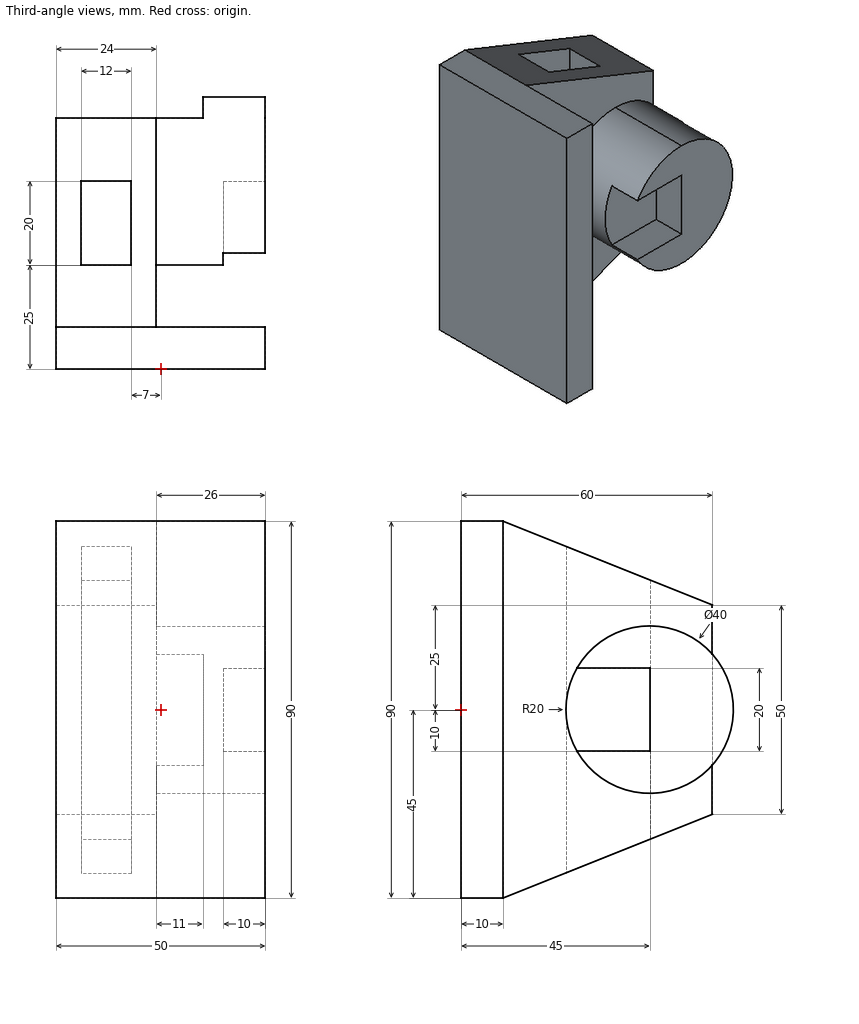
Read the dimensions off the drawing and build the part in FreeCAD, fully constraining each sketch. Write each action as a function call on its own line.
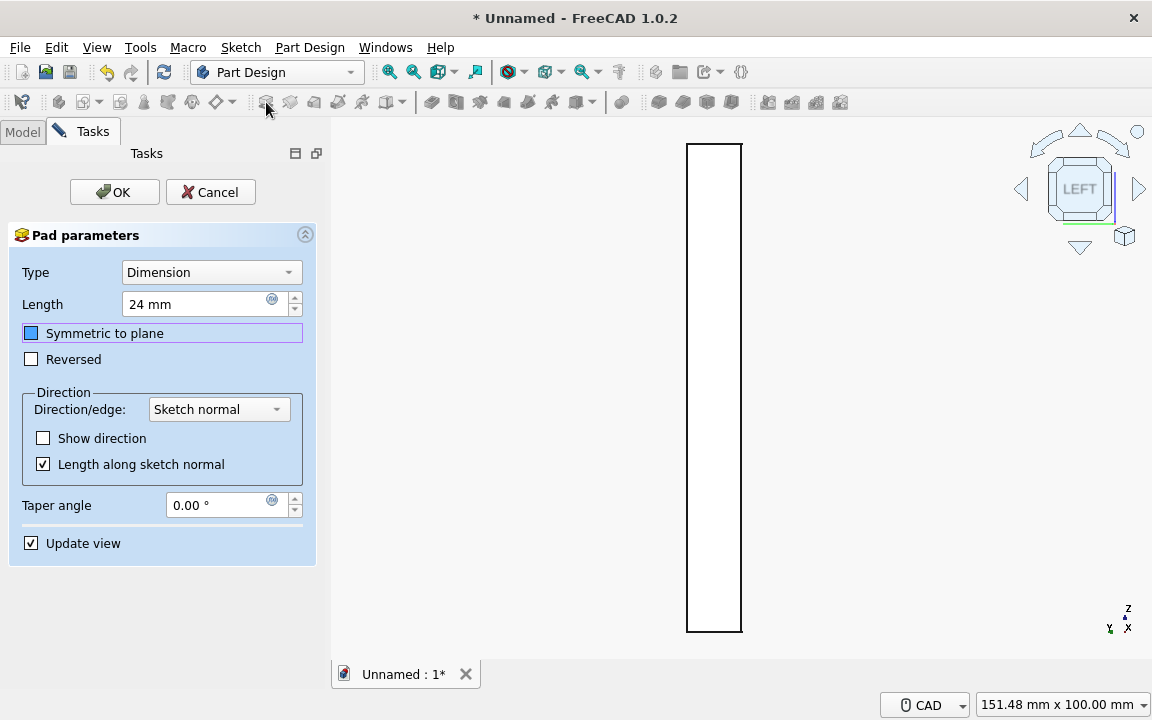
click(30, 359)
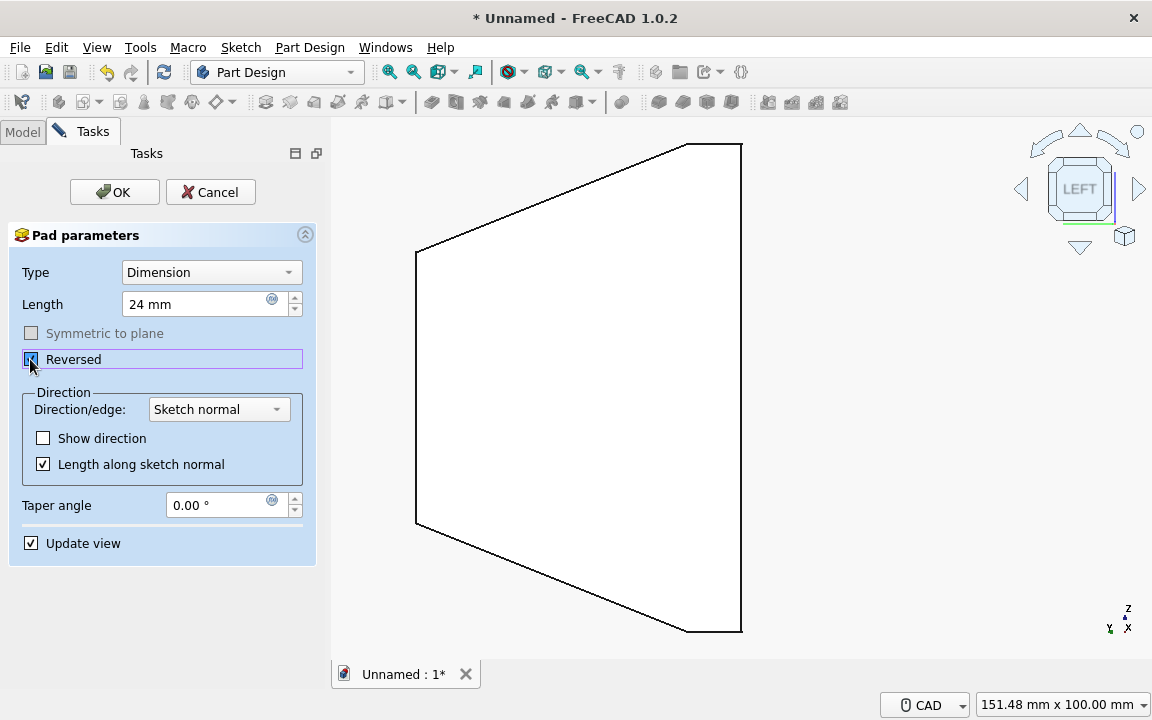
click(115, 192)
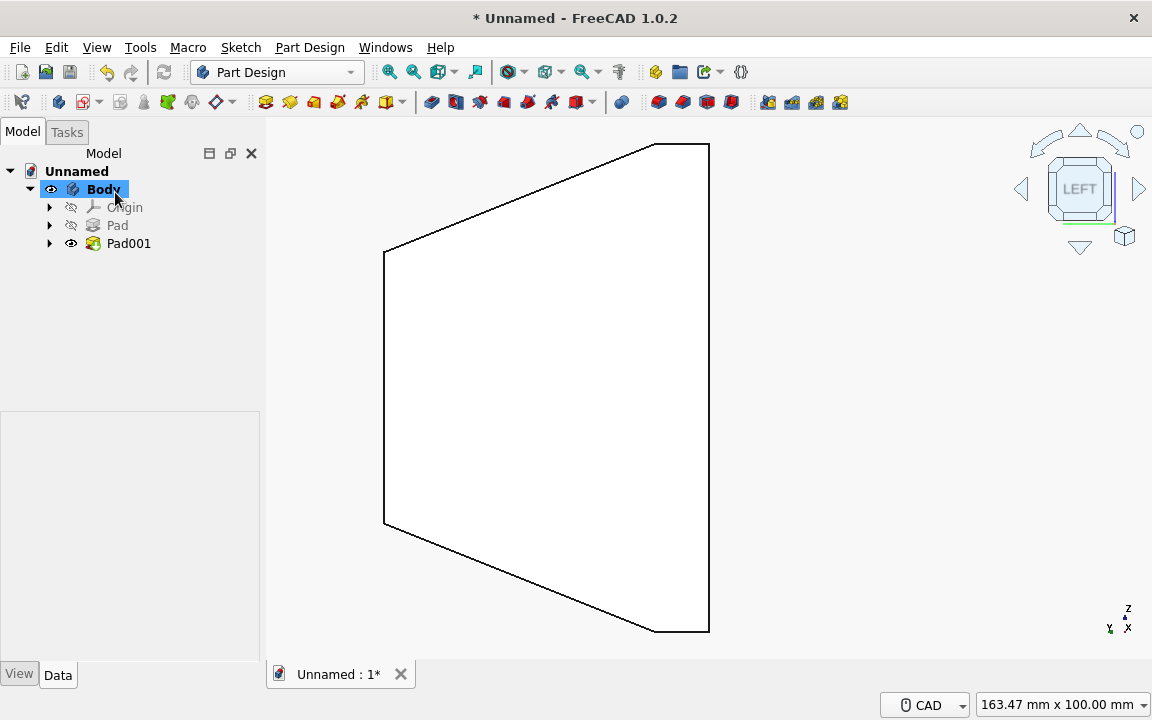
key(5)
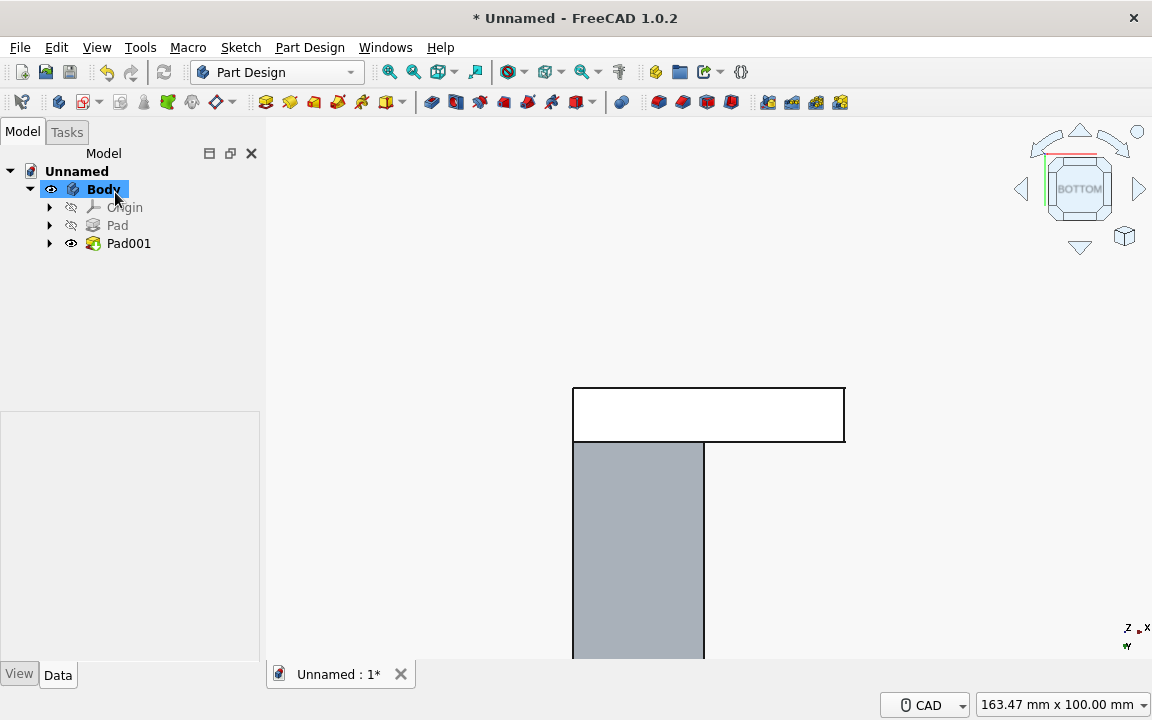
click(390, 72)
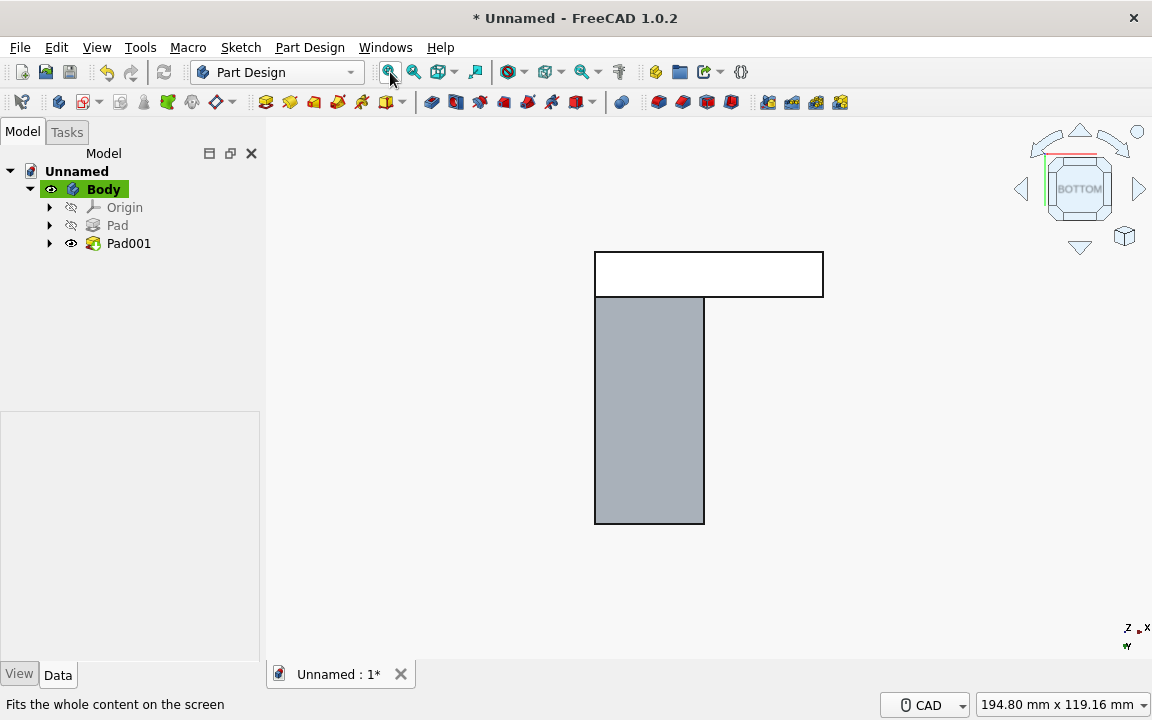
click(774, 273)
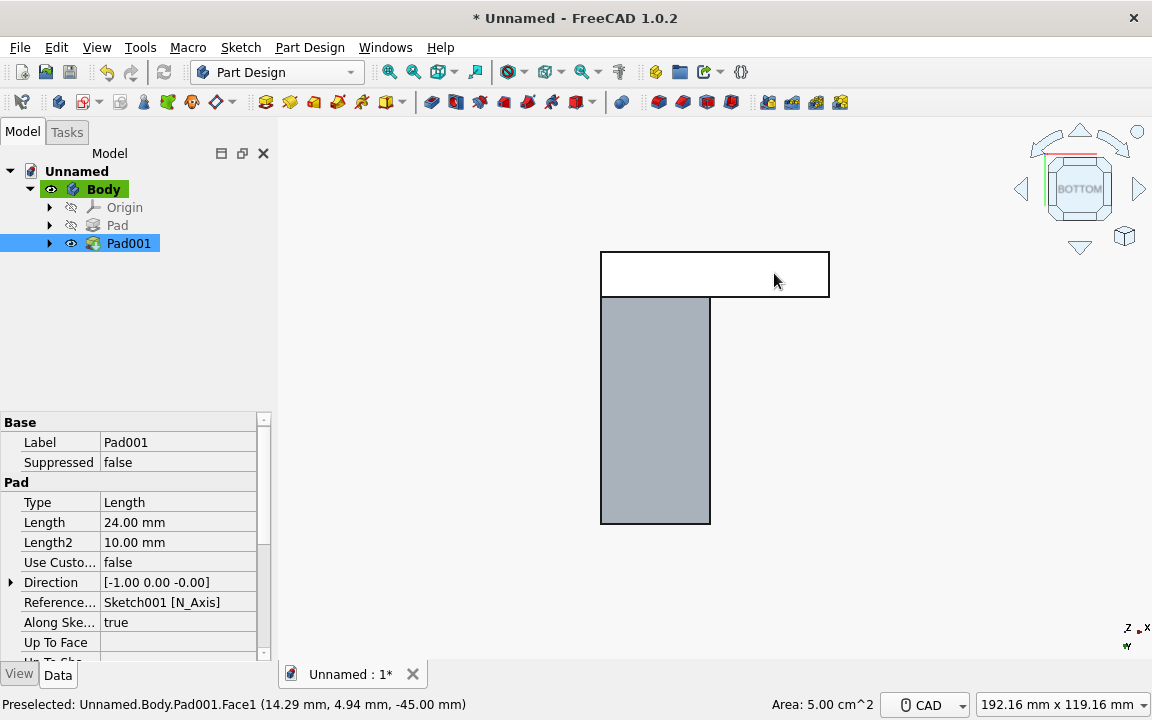
click(84, 102)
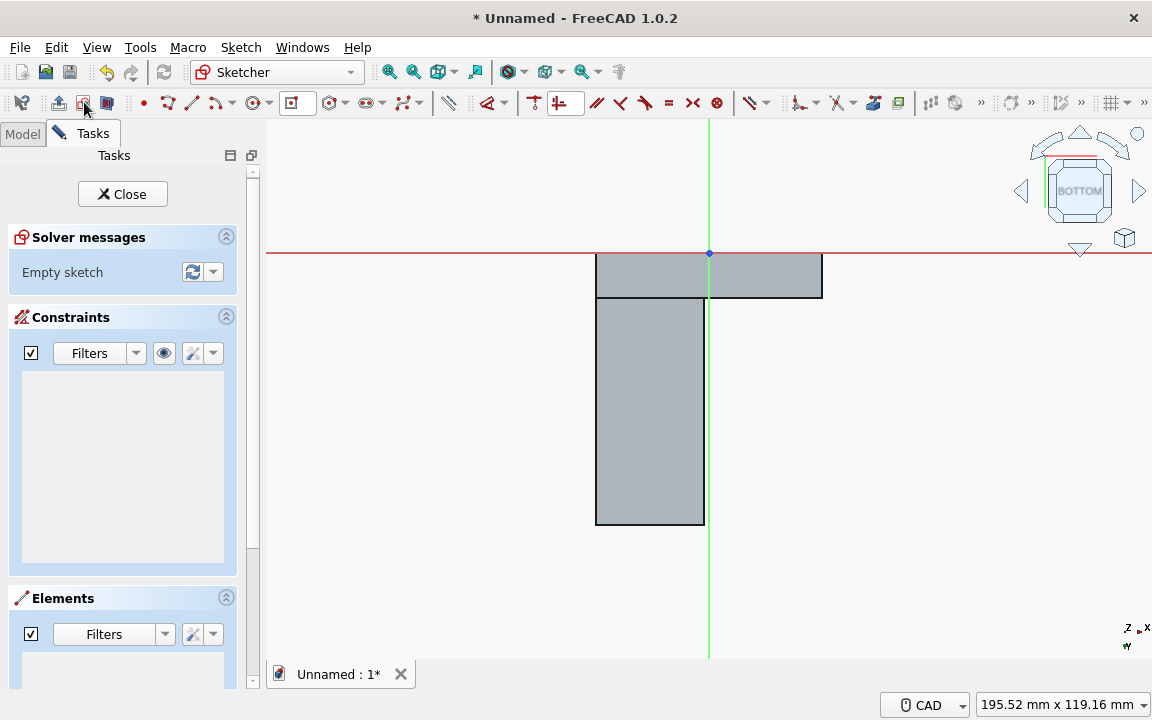
scroll(697, 314, up, 3)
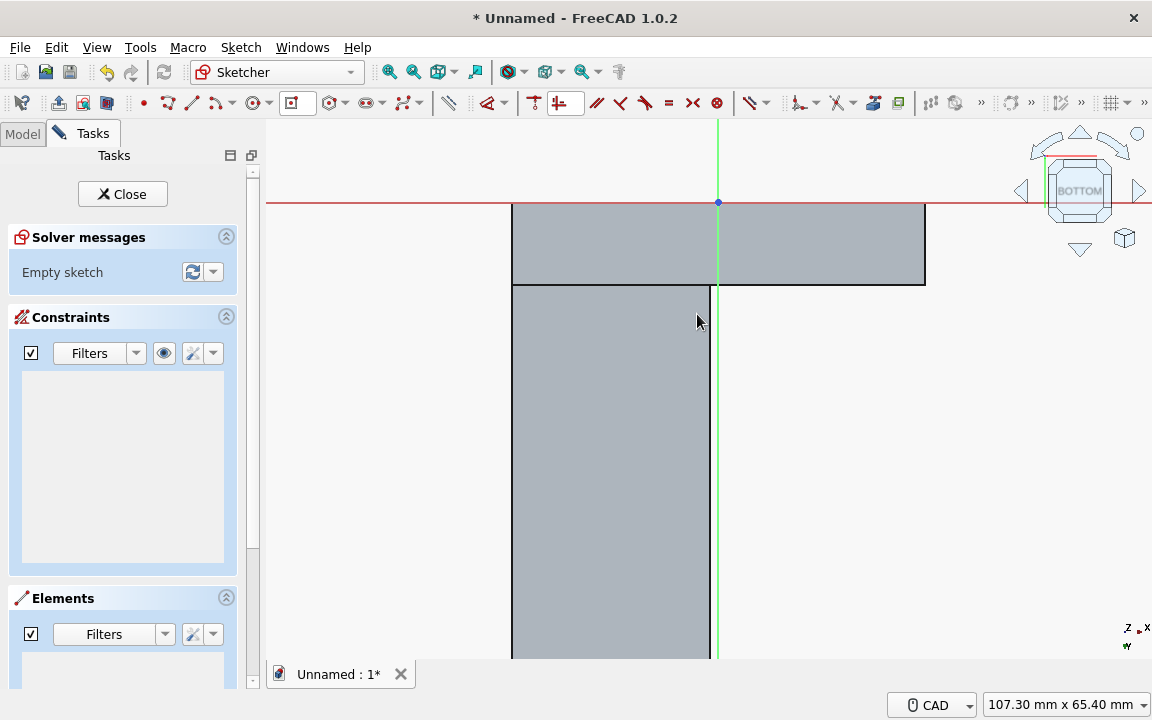
key(g)
key(r)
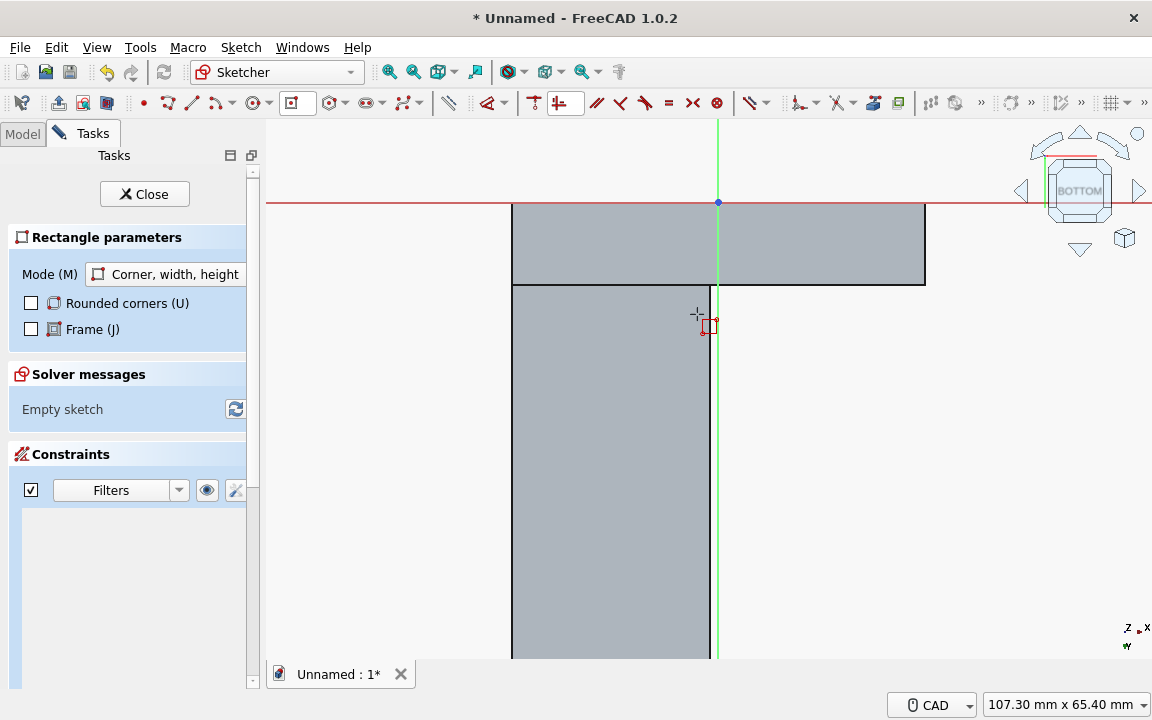
click(562, 409)
move(661, 574)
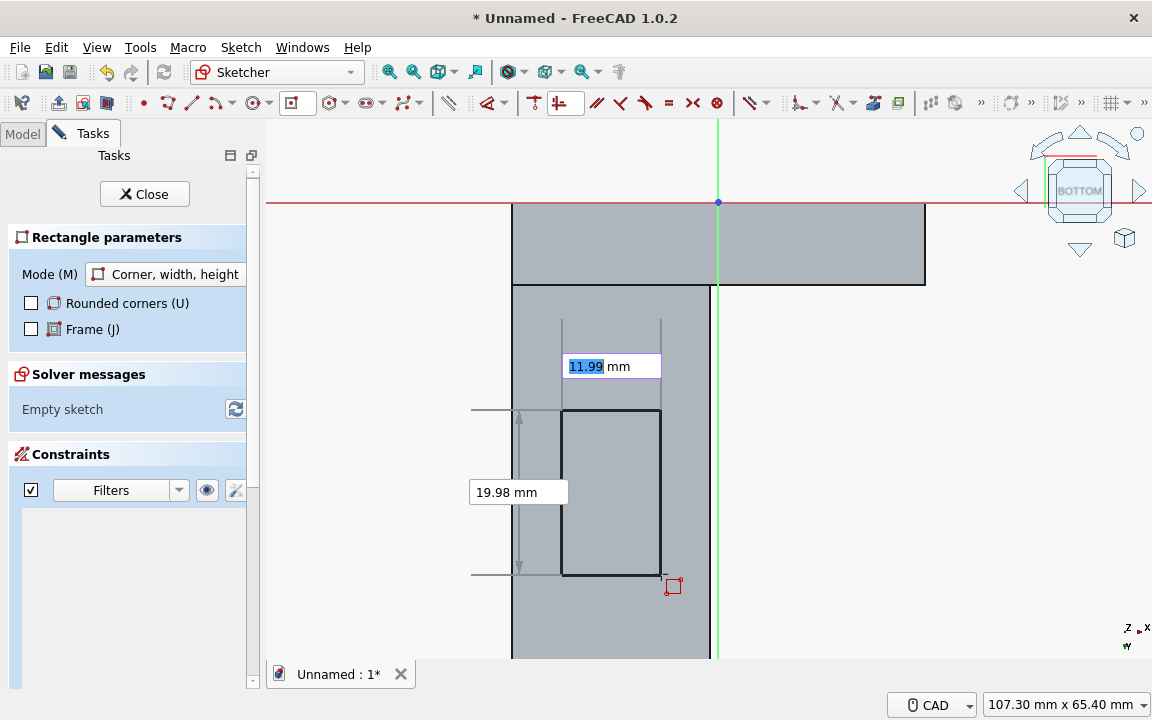
text(12)
key(Tab)
text(20)
key(Return)
key(Escape)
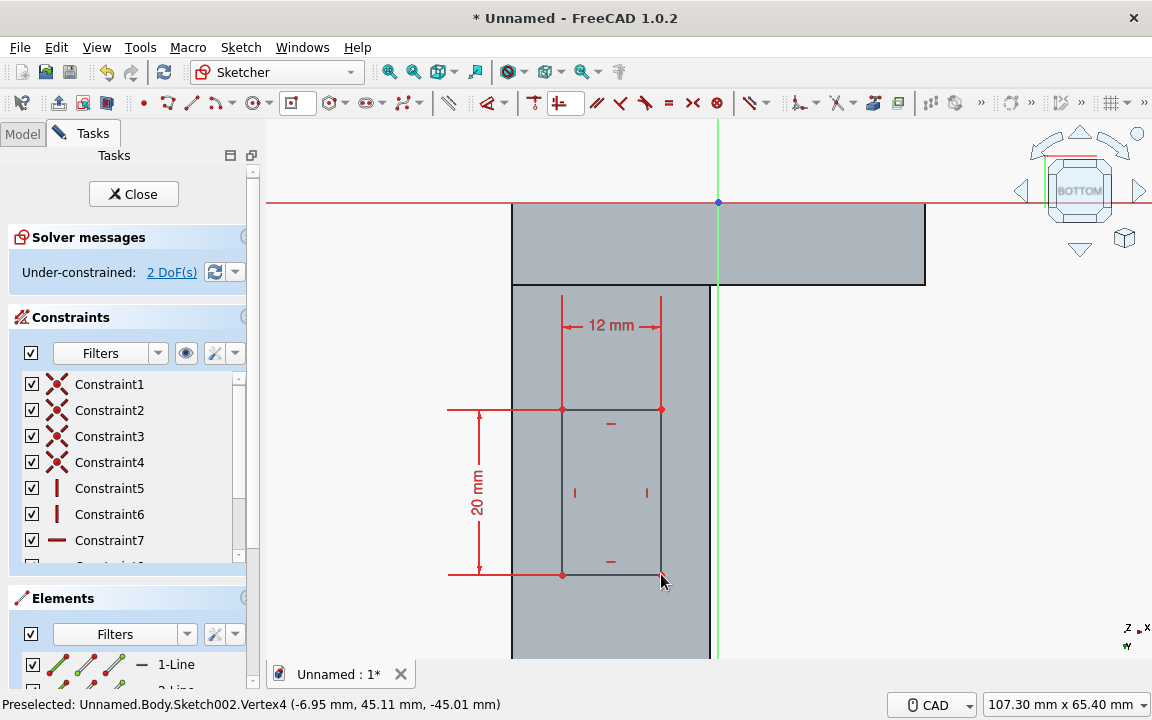
click(488, 104)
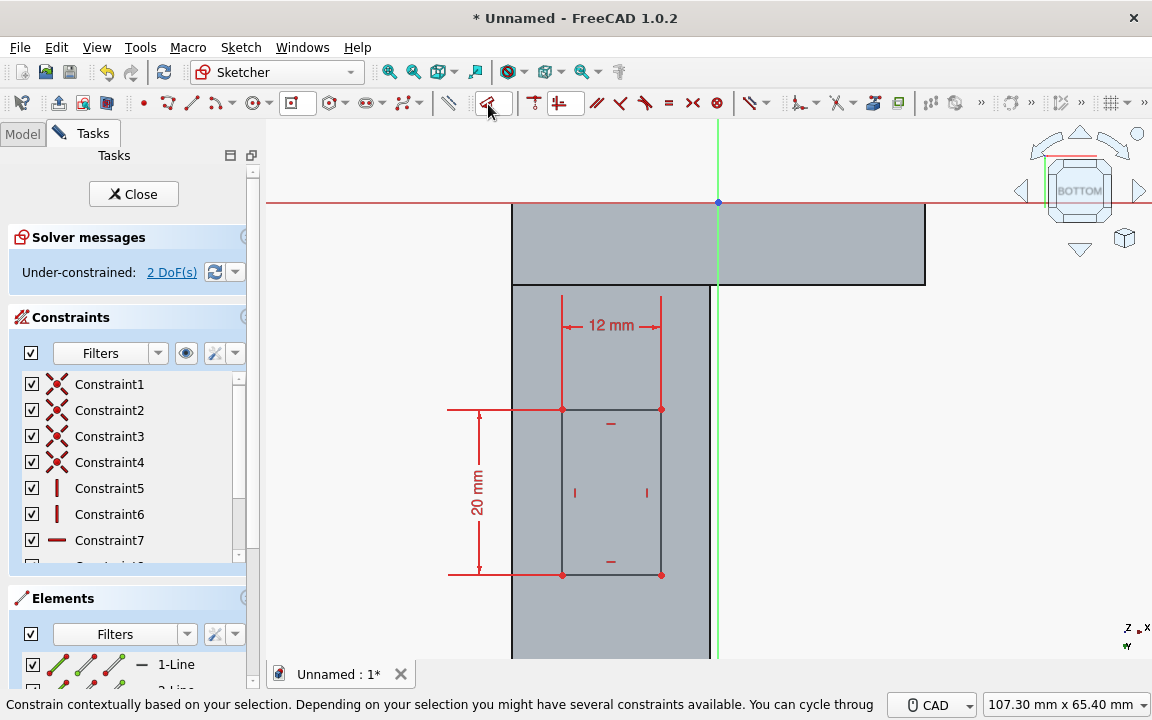
click(661, 575)
click(690, 609)